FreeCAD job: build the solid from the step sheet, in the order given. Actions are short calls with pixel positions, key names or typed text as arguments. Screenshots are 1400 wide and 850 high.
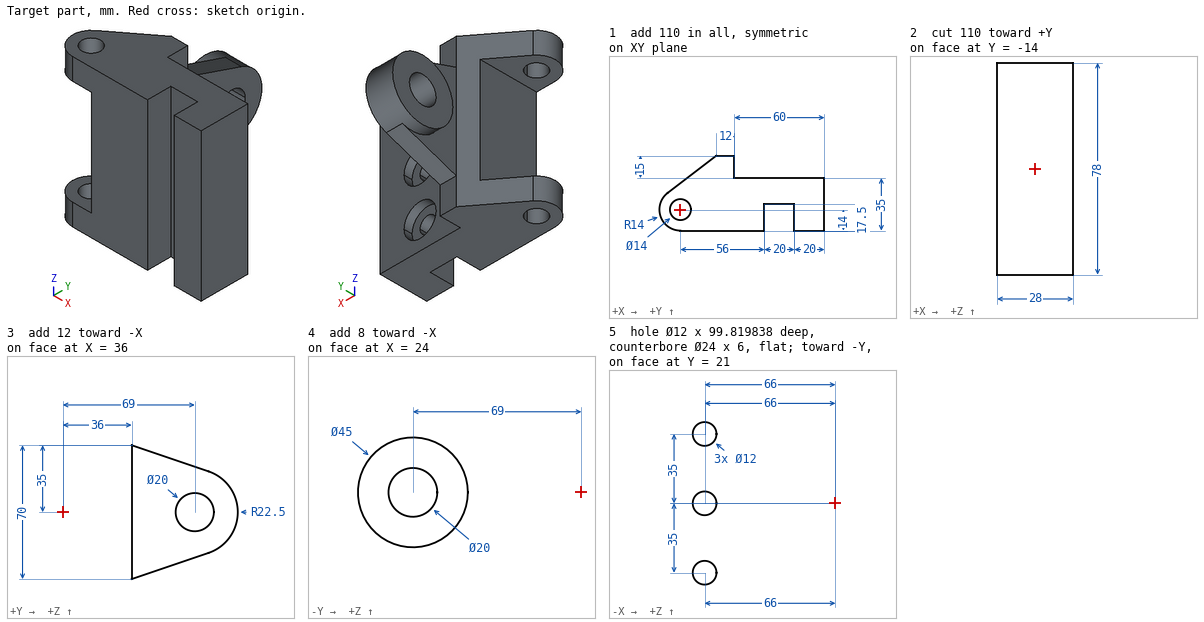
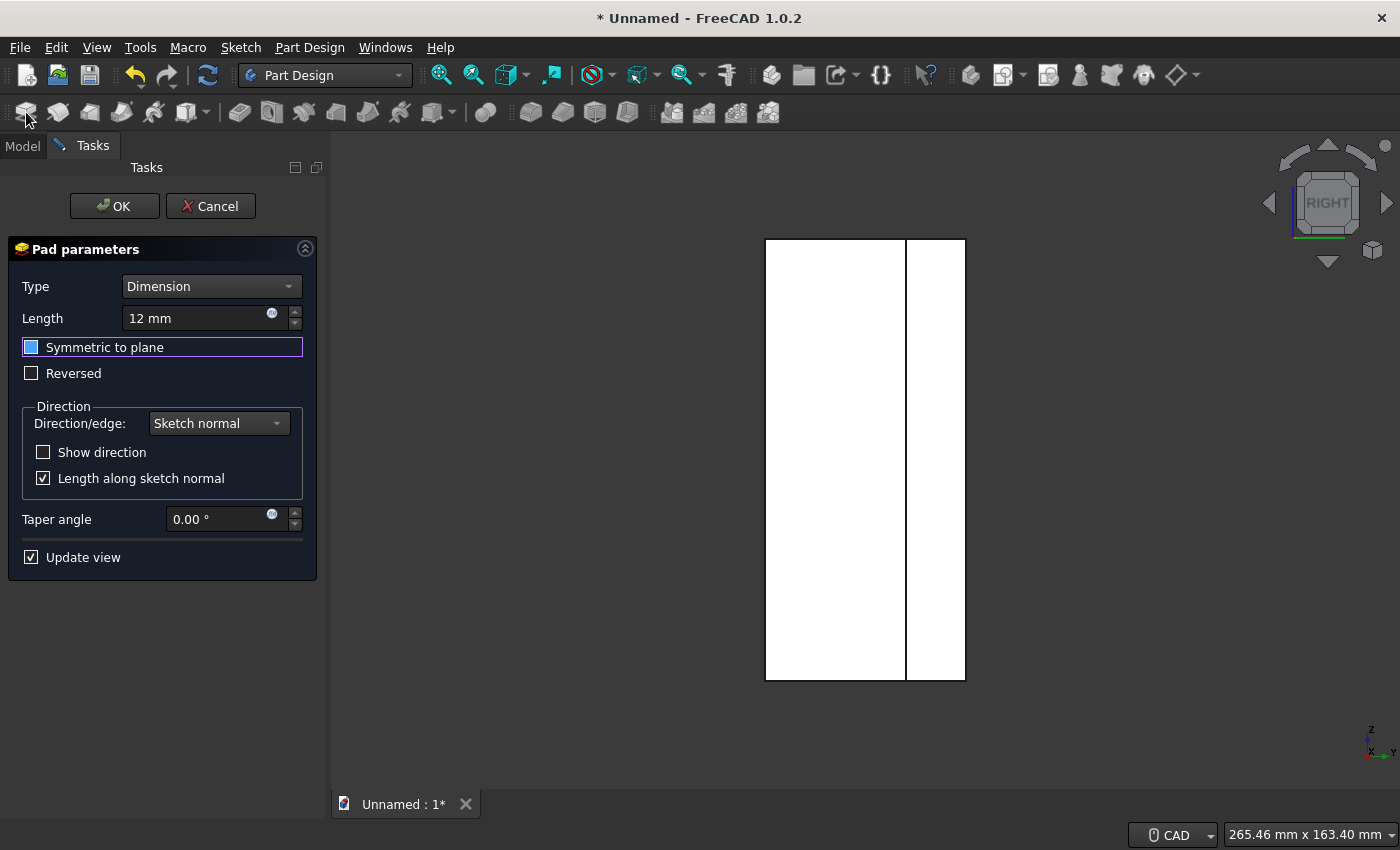
click(30, 373)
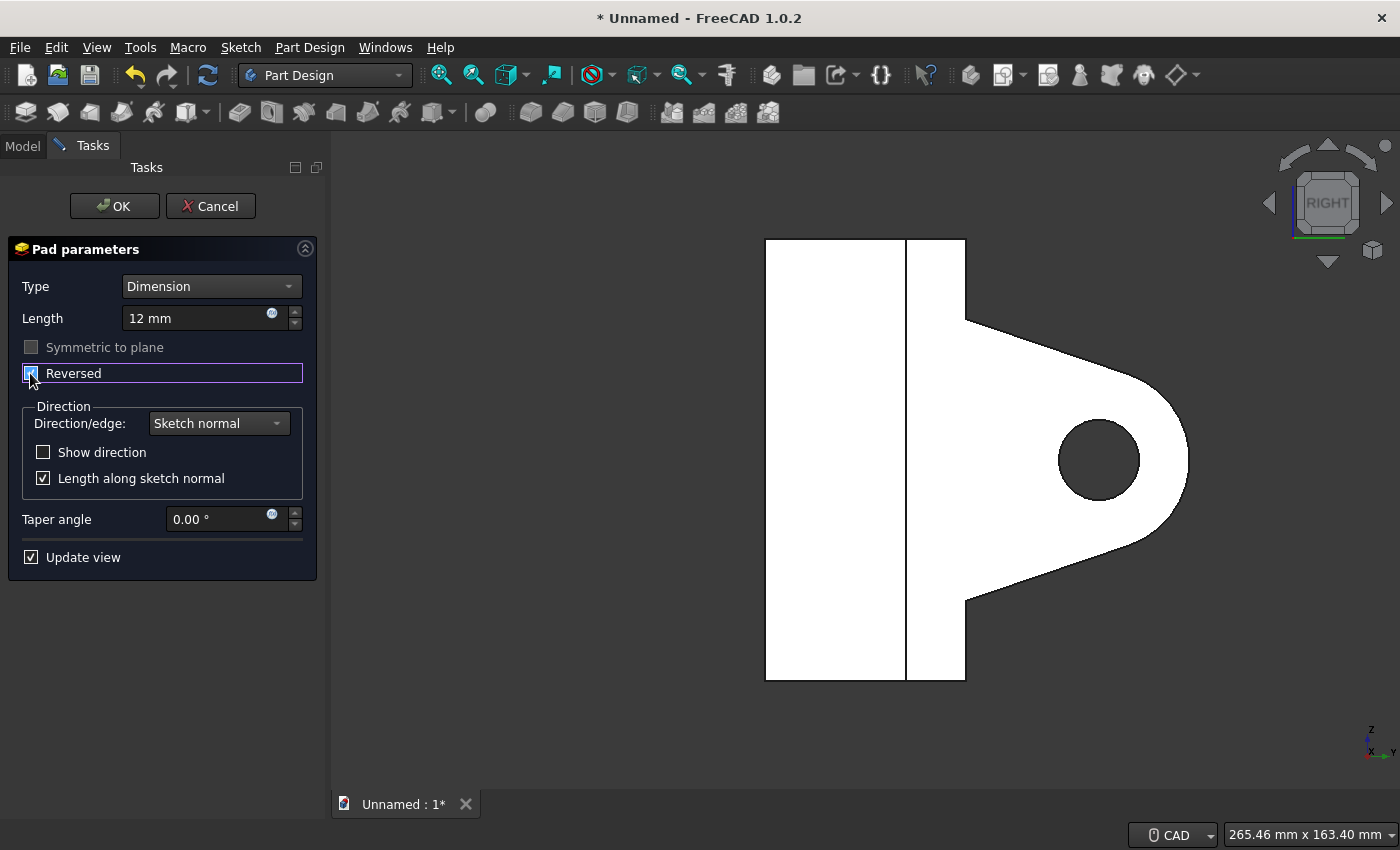
click(115, 206)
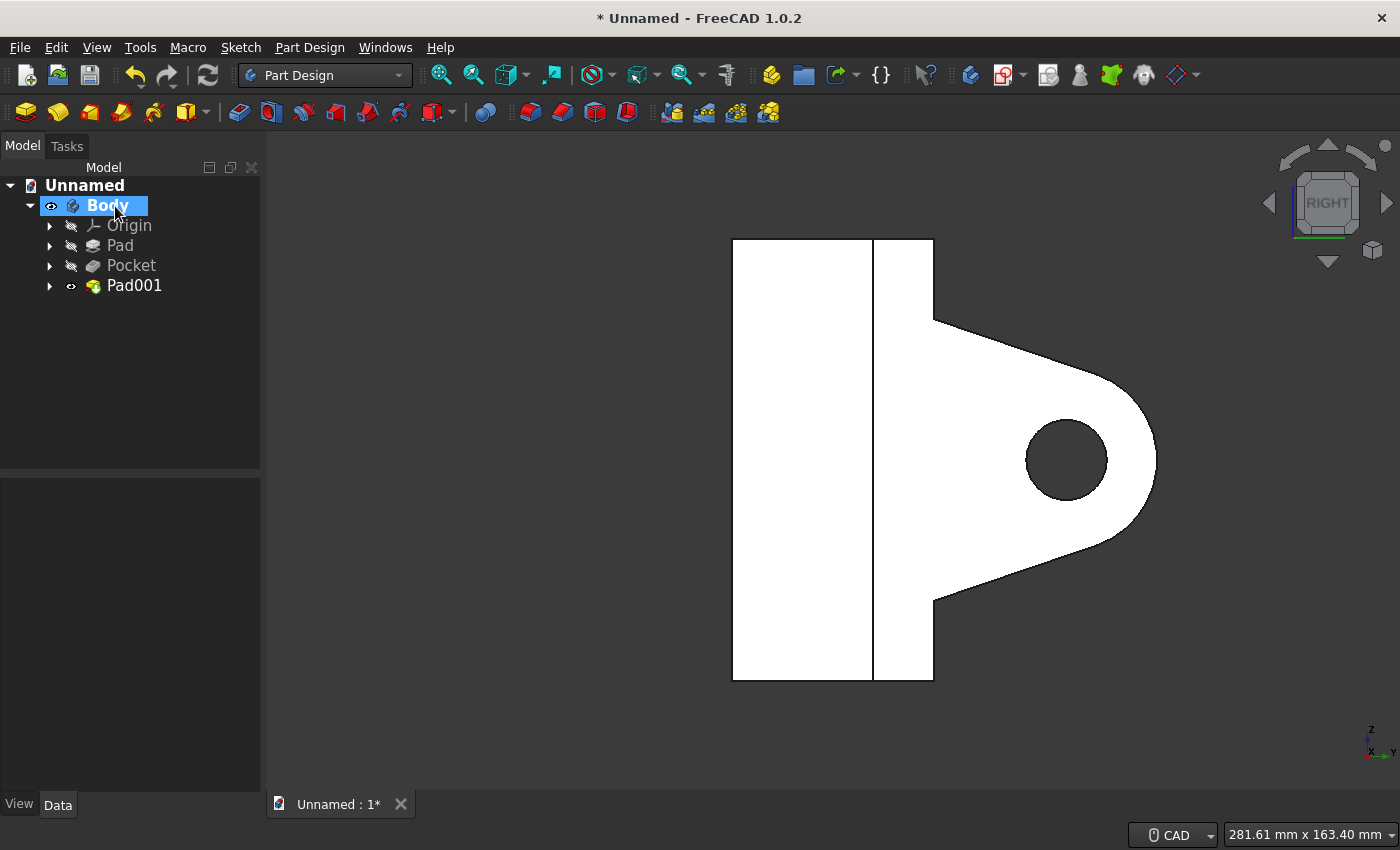
key(6)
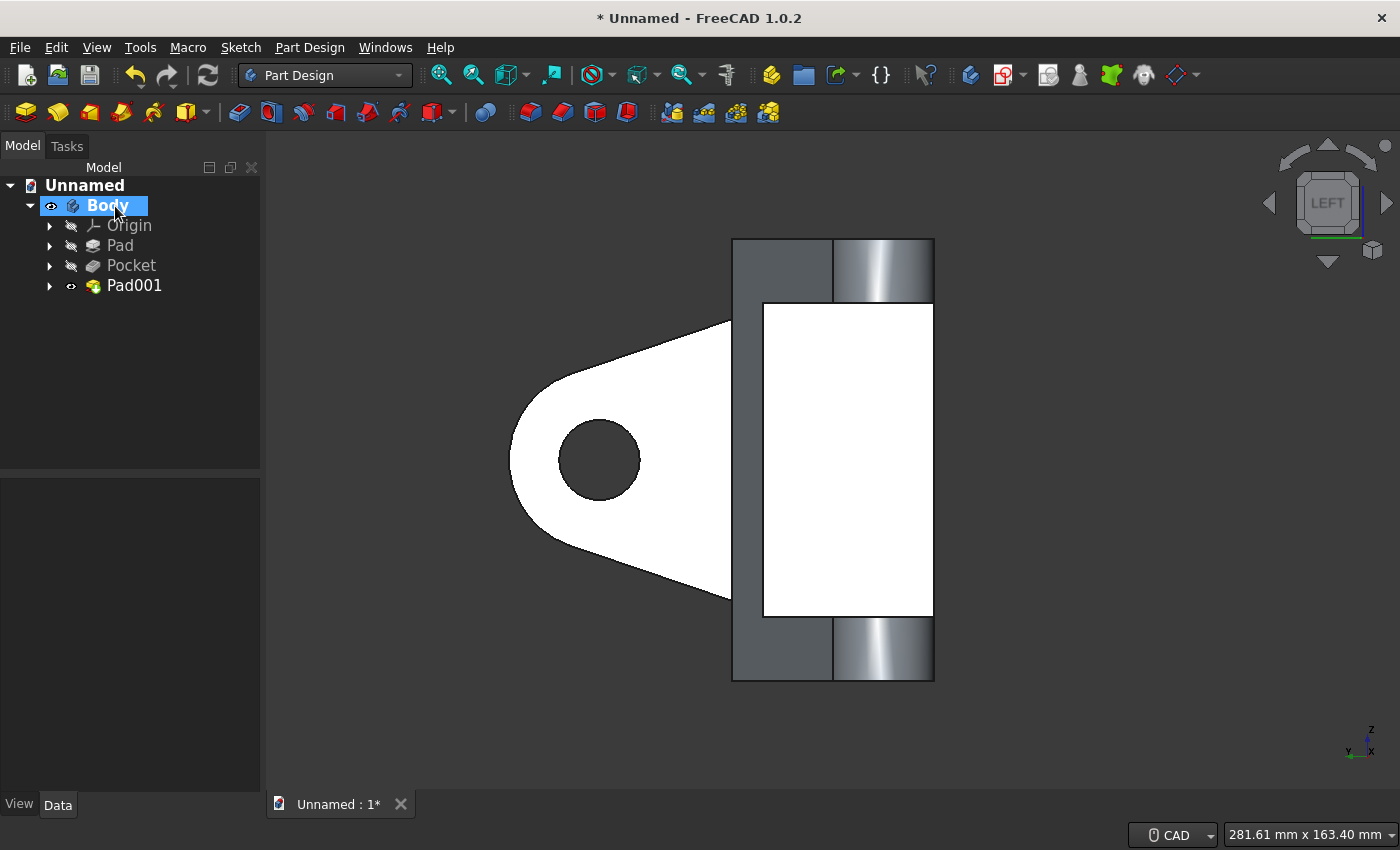
click(684, 419)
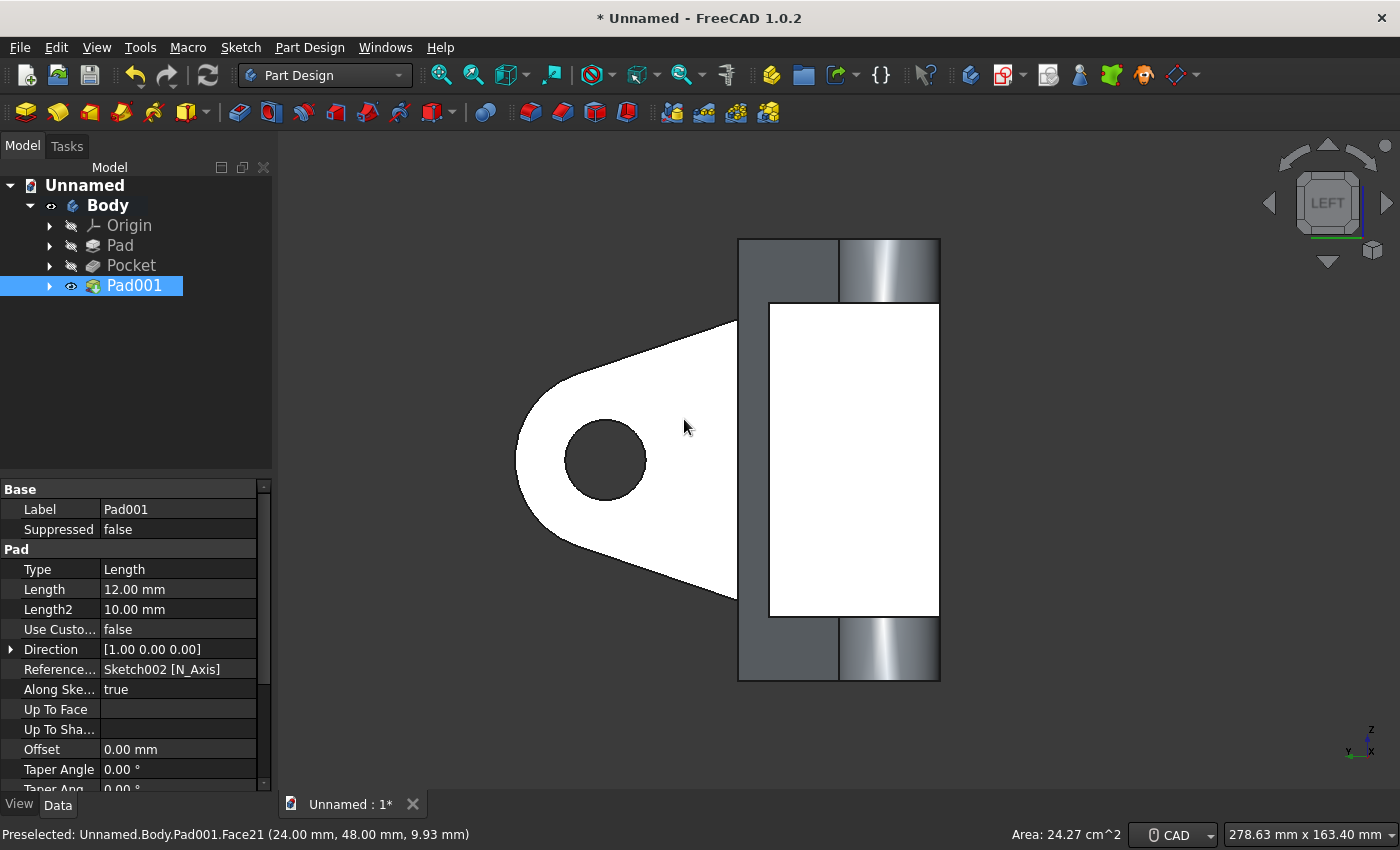
click(1004, 76)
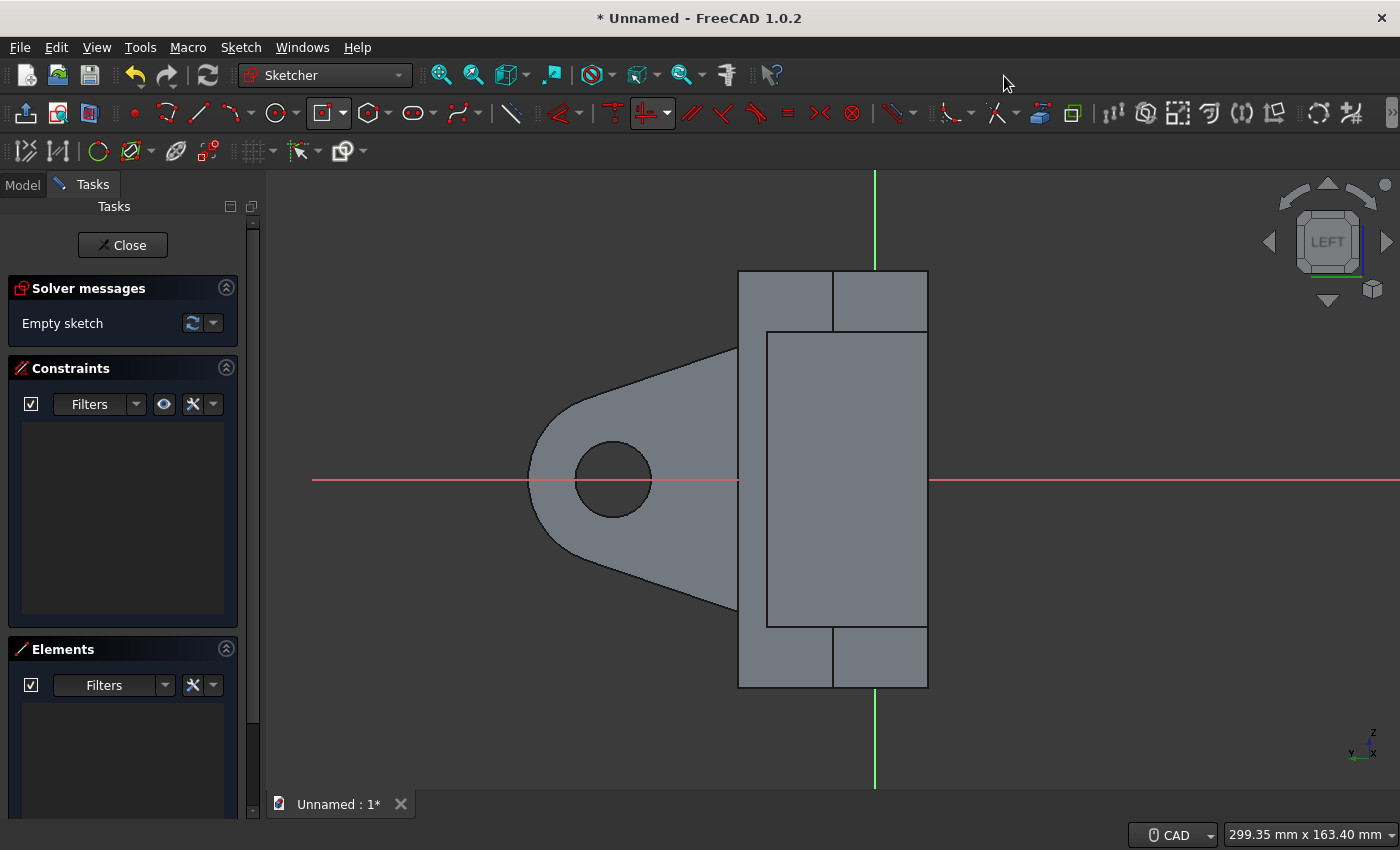
scroll(625, 480, up, 3)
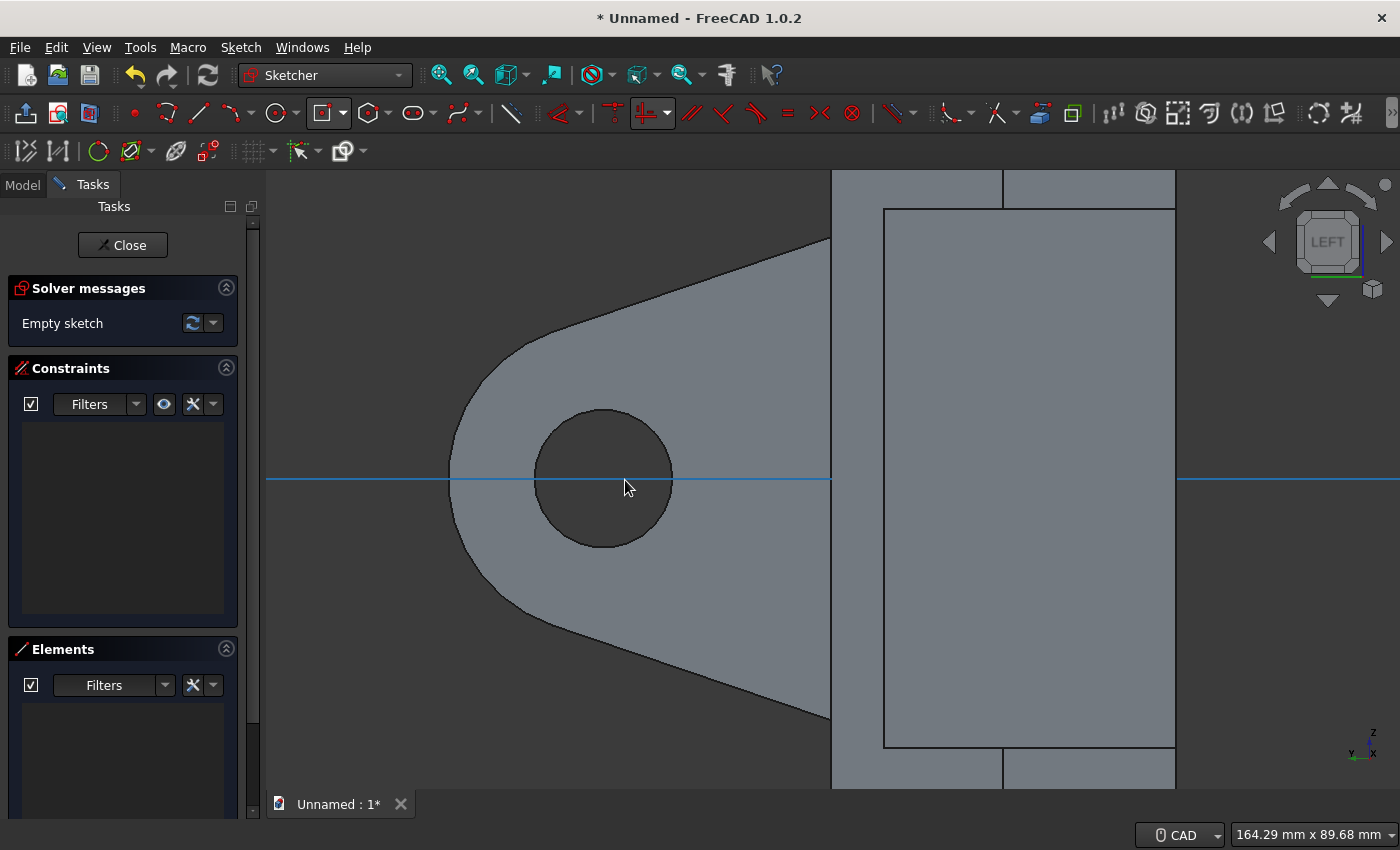
click(276, 114)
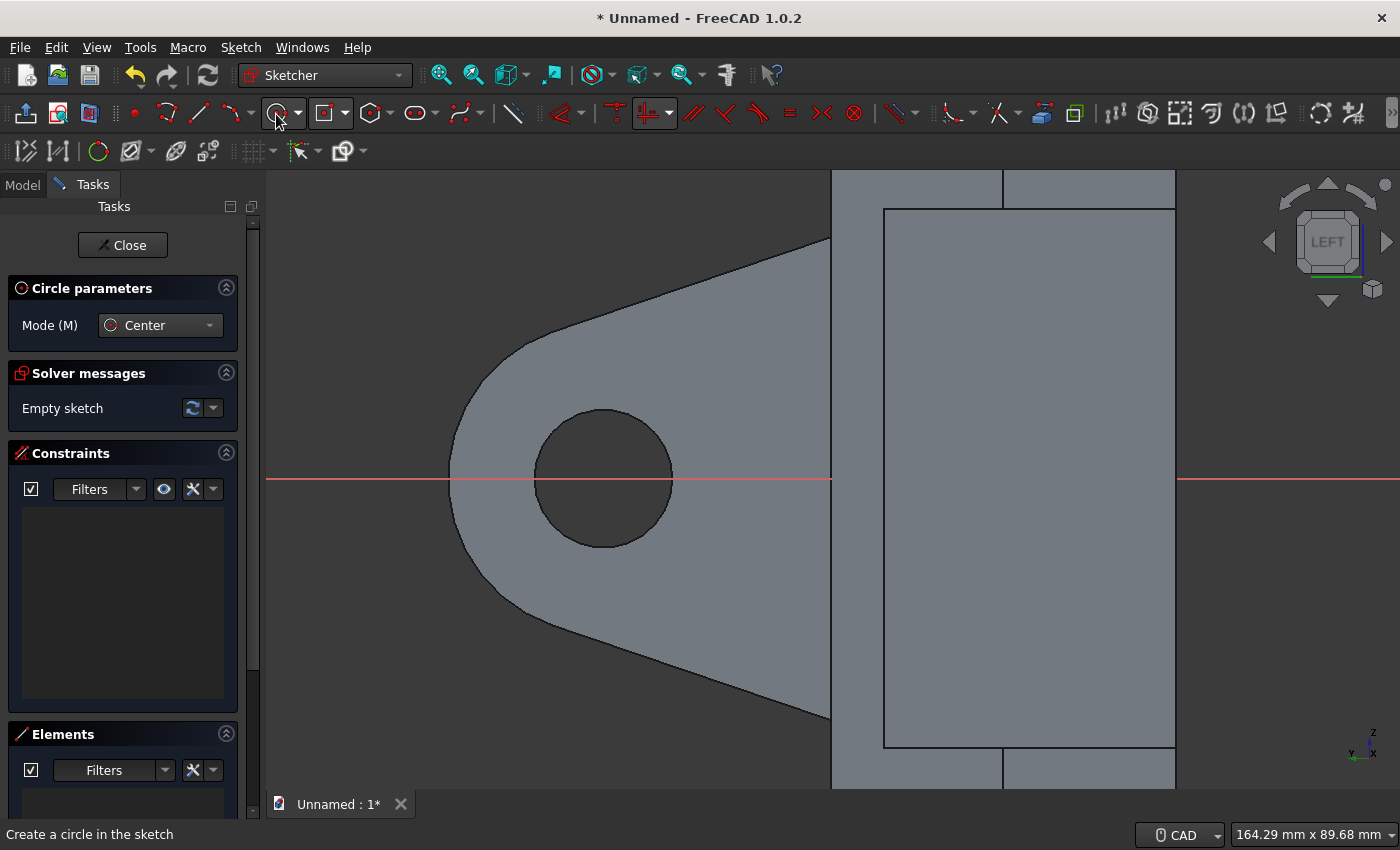
click(603, 479)
click(713, 369)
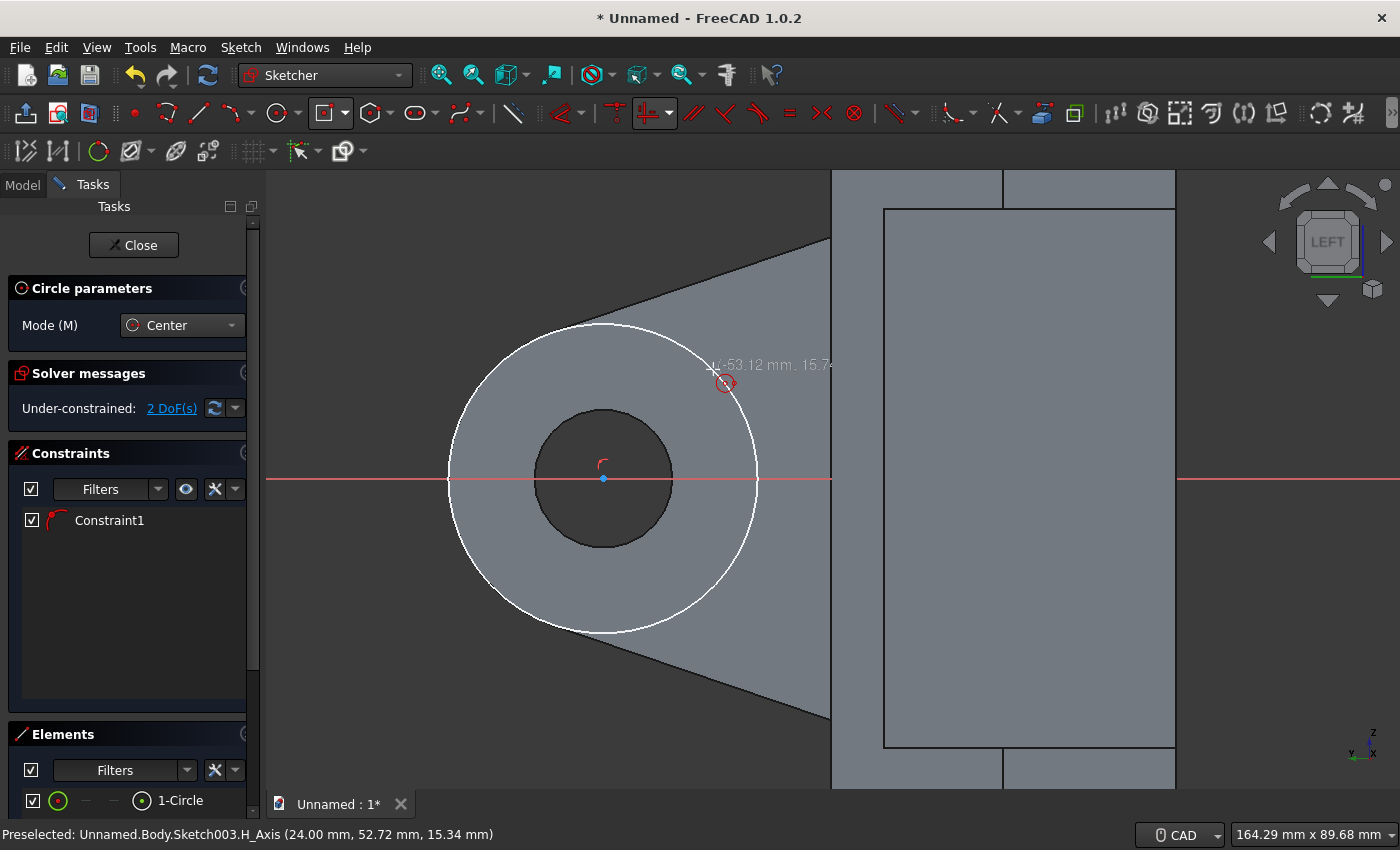
click(603, 479)
click(652, 430)
key(Escape)